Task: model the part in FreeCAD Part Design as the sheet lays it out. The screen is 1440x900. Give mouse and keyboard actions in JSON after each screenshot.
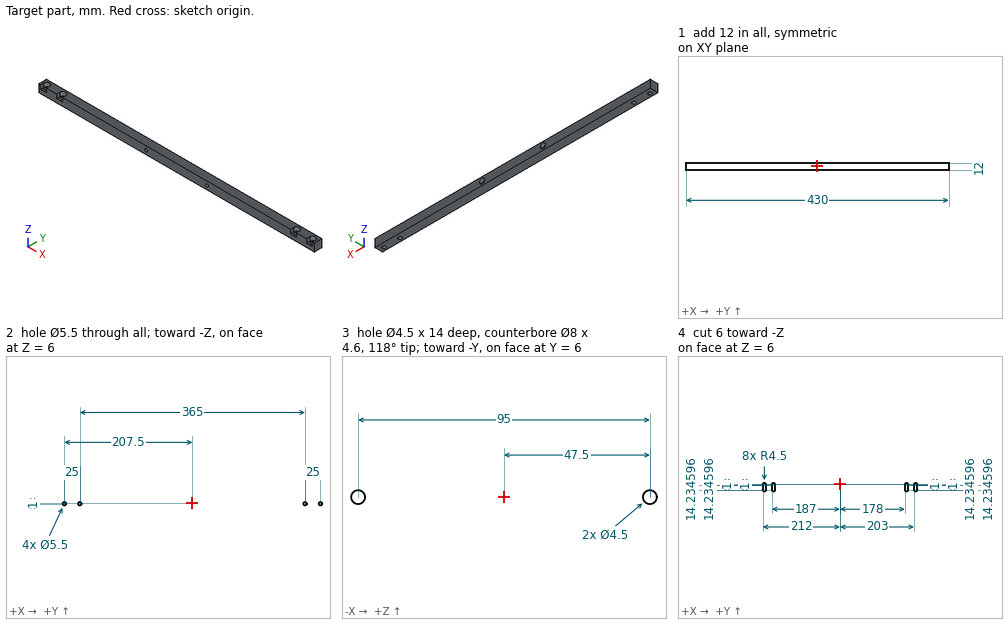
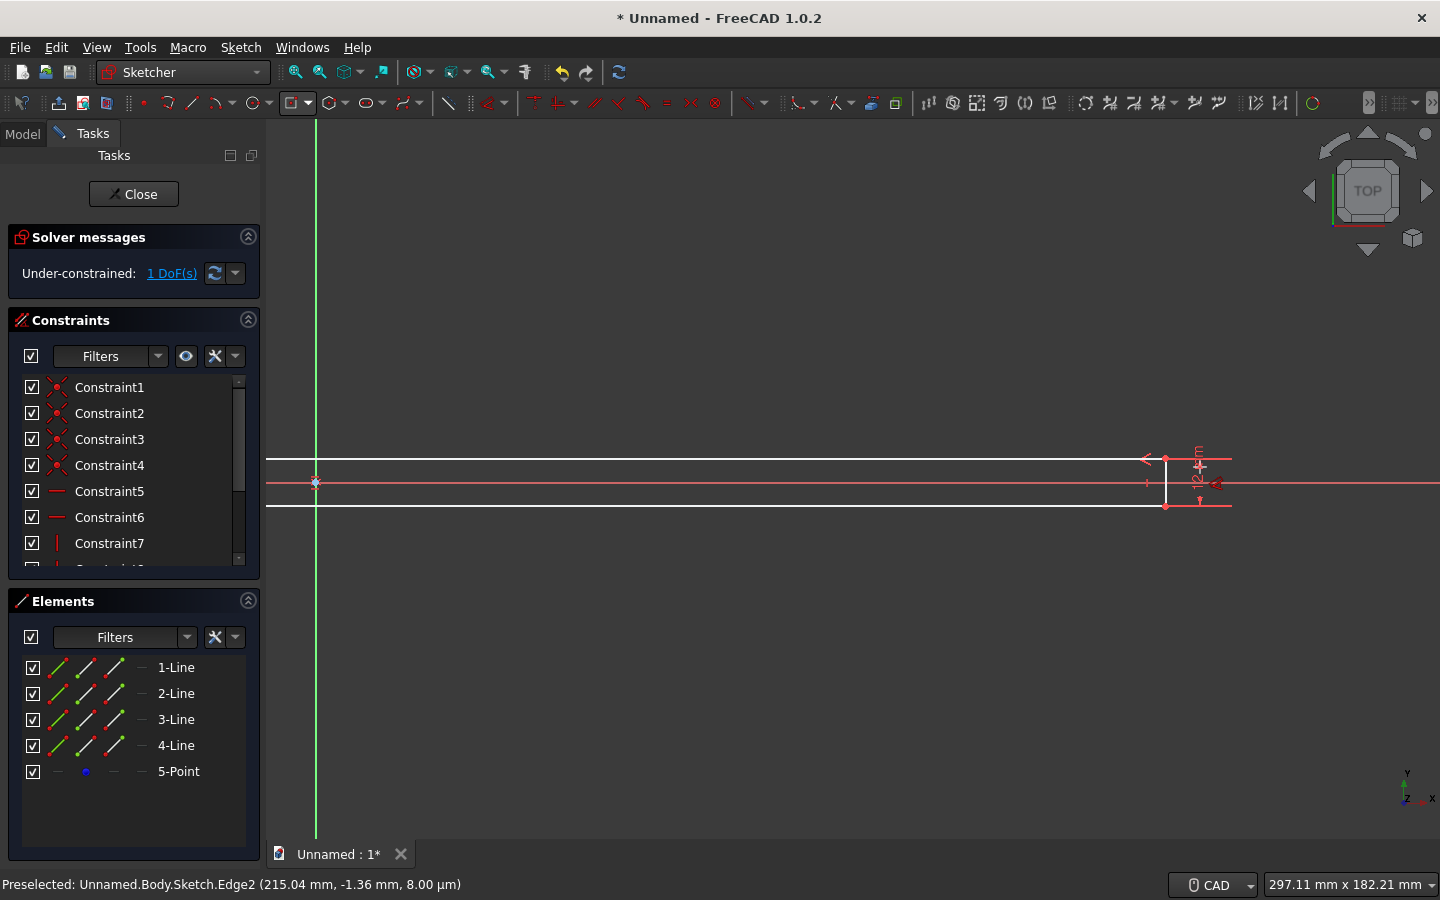
{"action": "left_click", "coordinate": [656, 506]}
{"action": "left_click", "coordinate": [730, 540]}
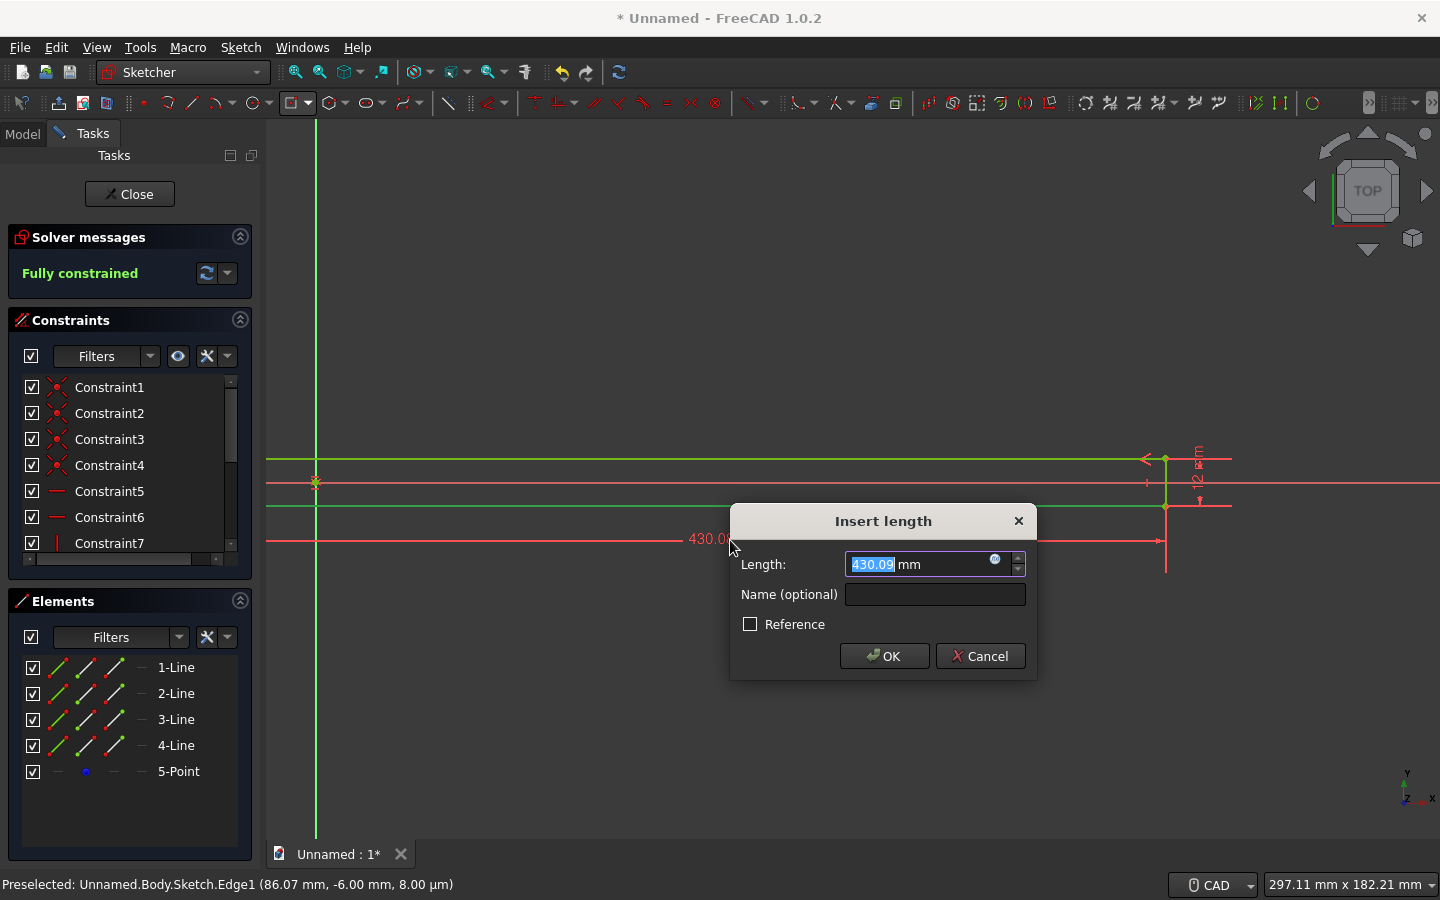
{"action": "type", "text": "430"}
{"action": "key", "text": "Return"}
{"action": "key", "text": "Escape"}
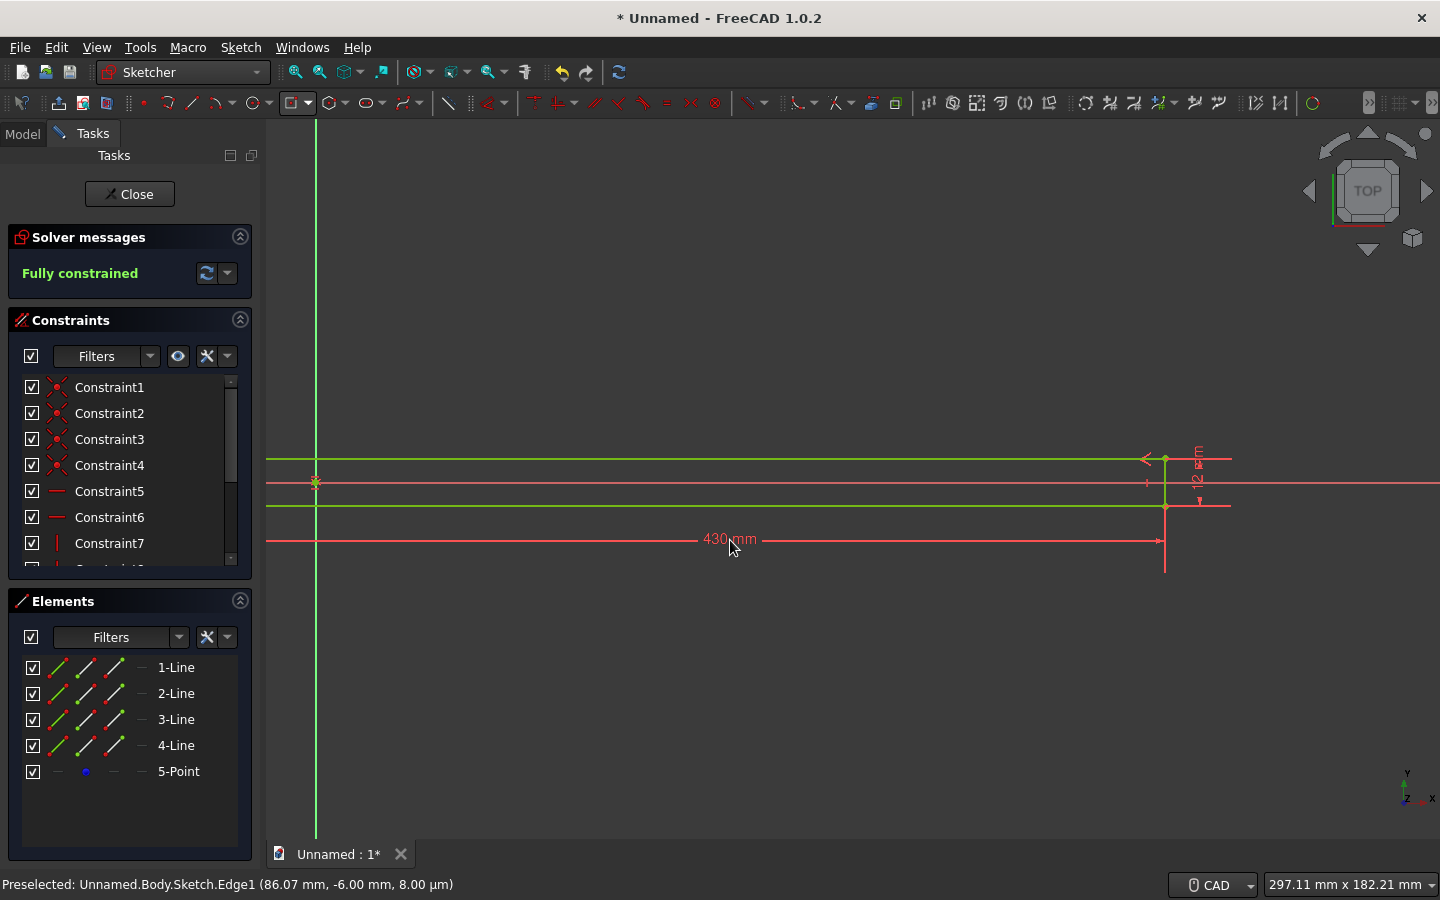
{"action": "left_click", "coordinate": [130, 194]}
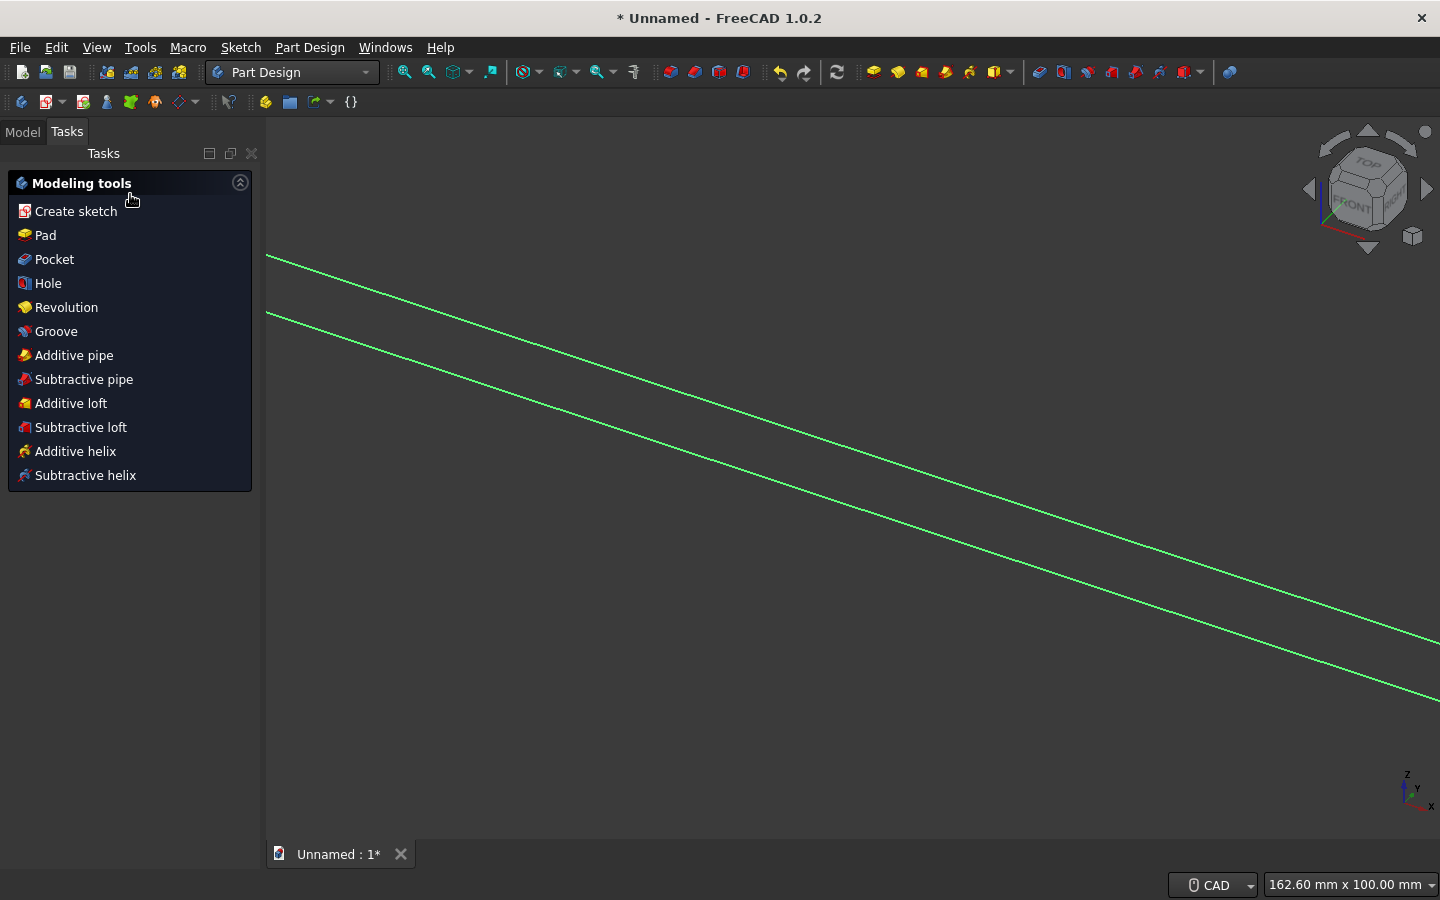
{"action": "left_click", "coordinate": [874, 72]}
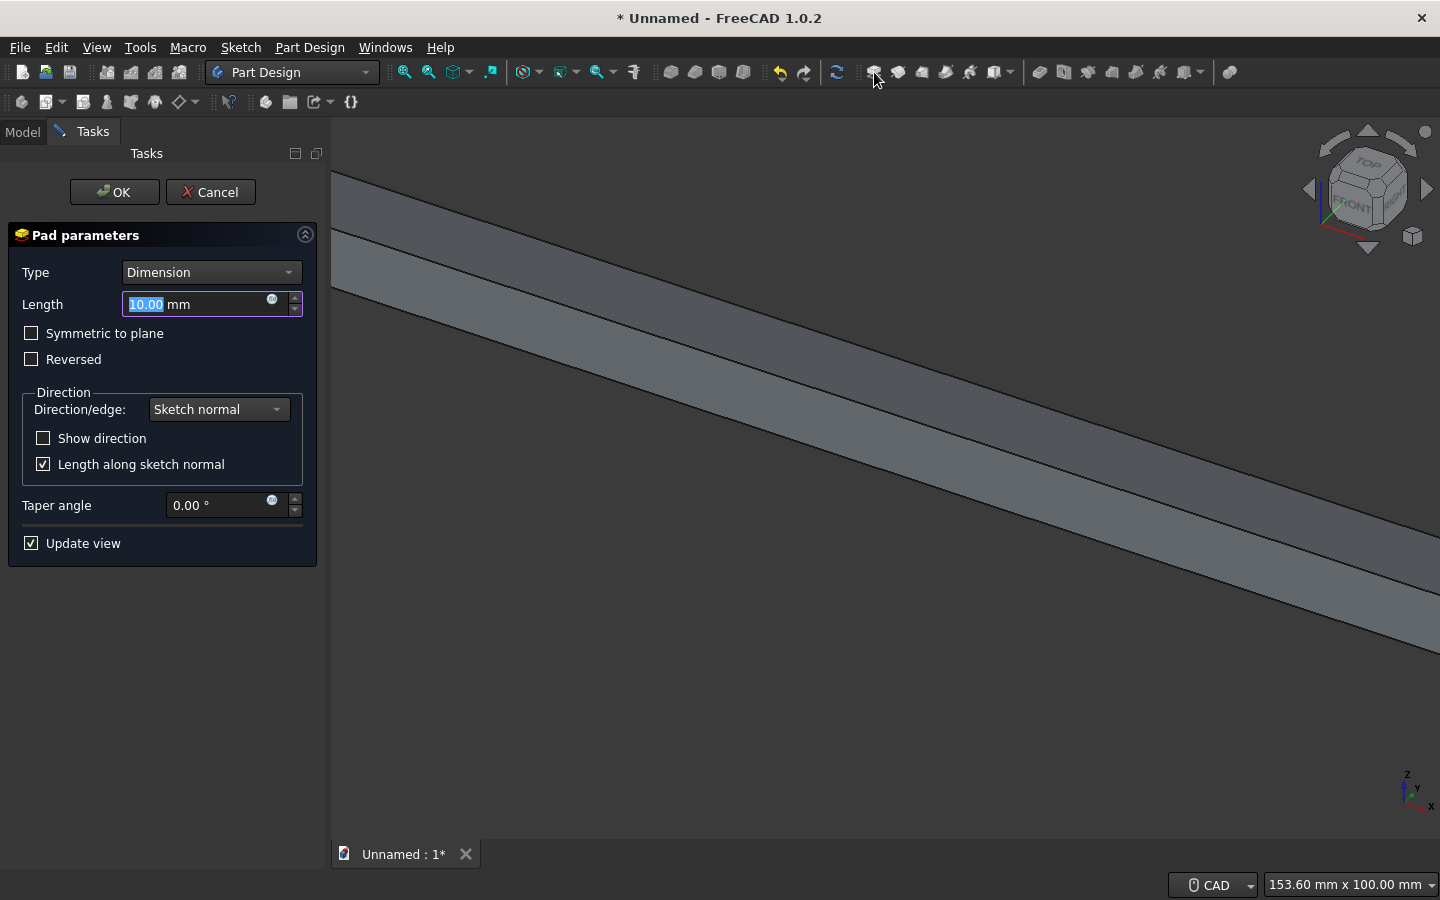
{"action": "type", "text": "12"}
{"action": "key", "text": "Tab"}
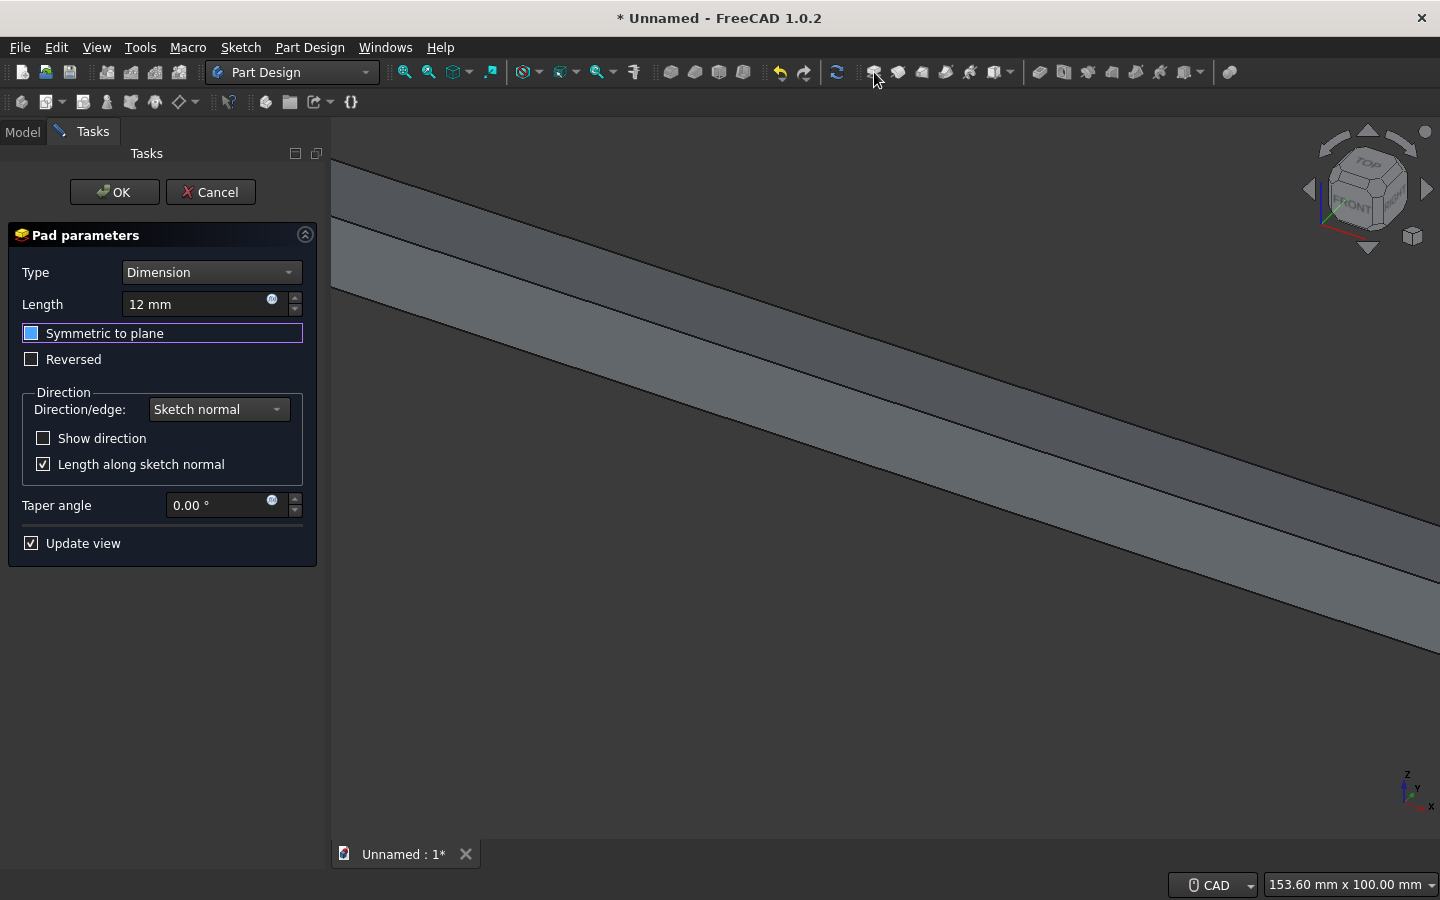
{"action": "left_click", "coordinate": [30, 333]}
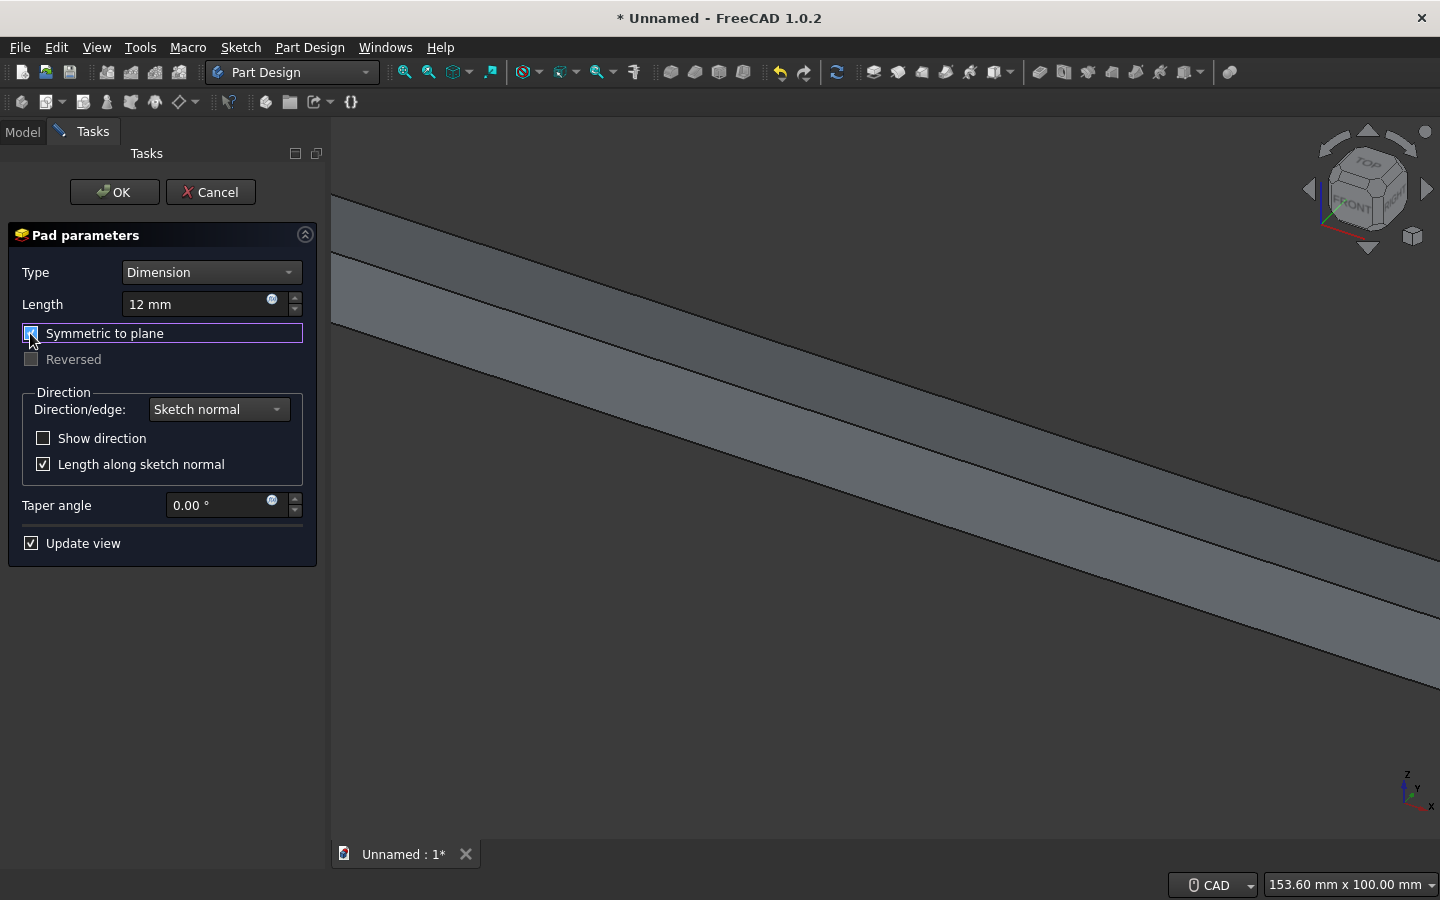
{"action": "left_click", "coordinate": [115, 192]}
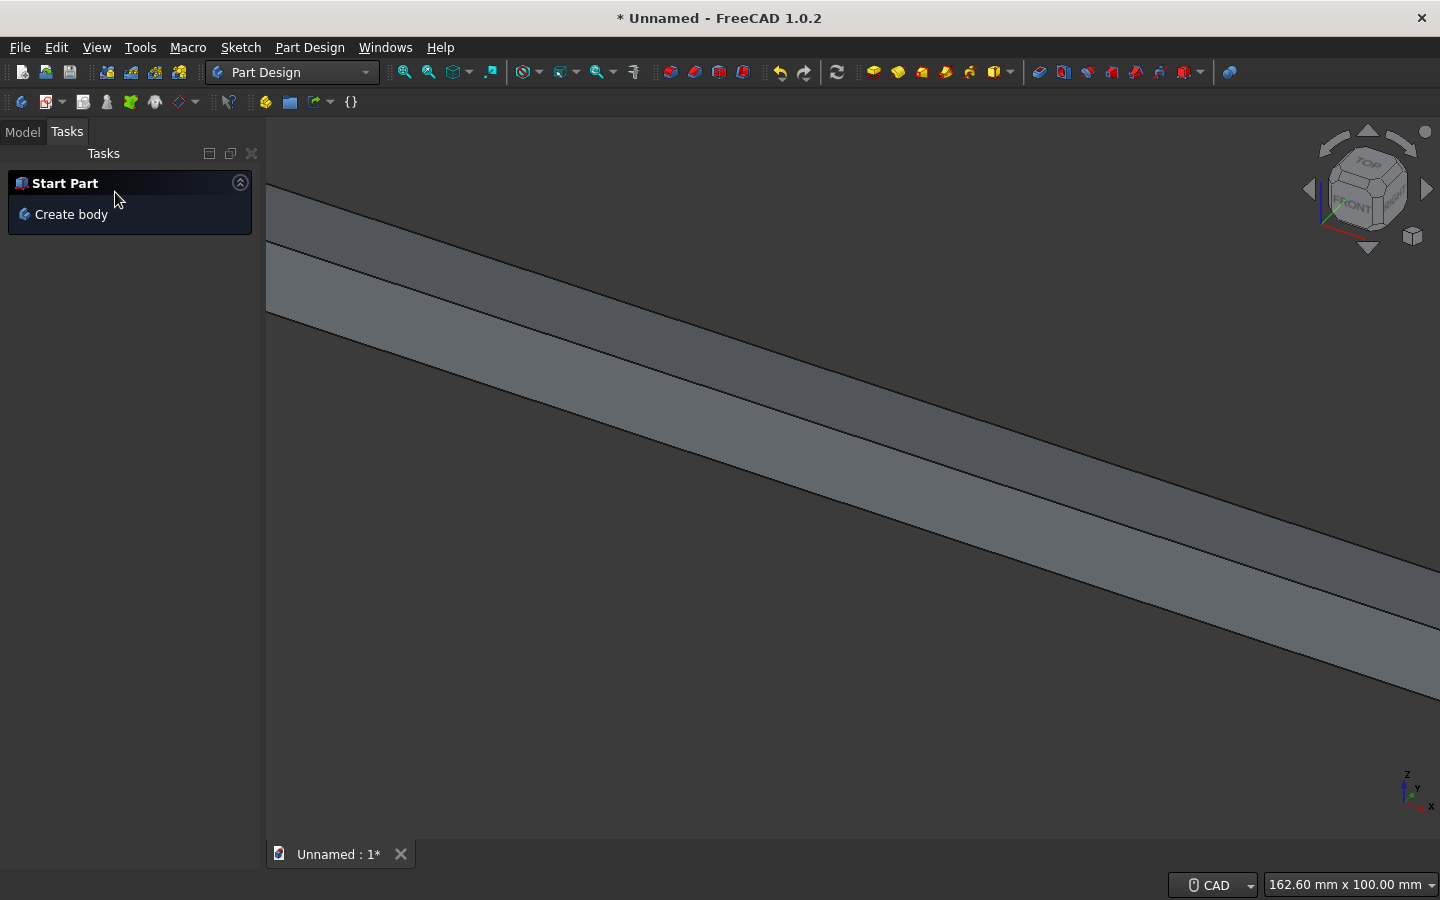
{"action": "key", "text": "v f"}